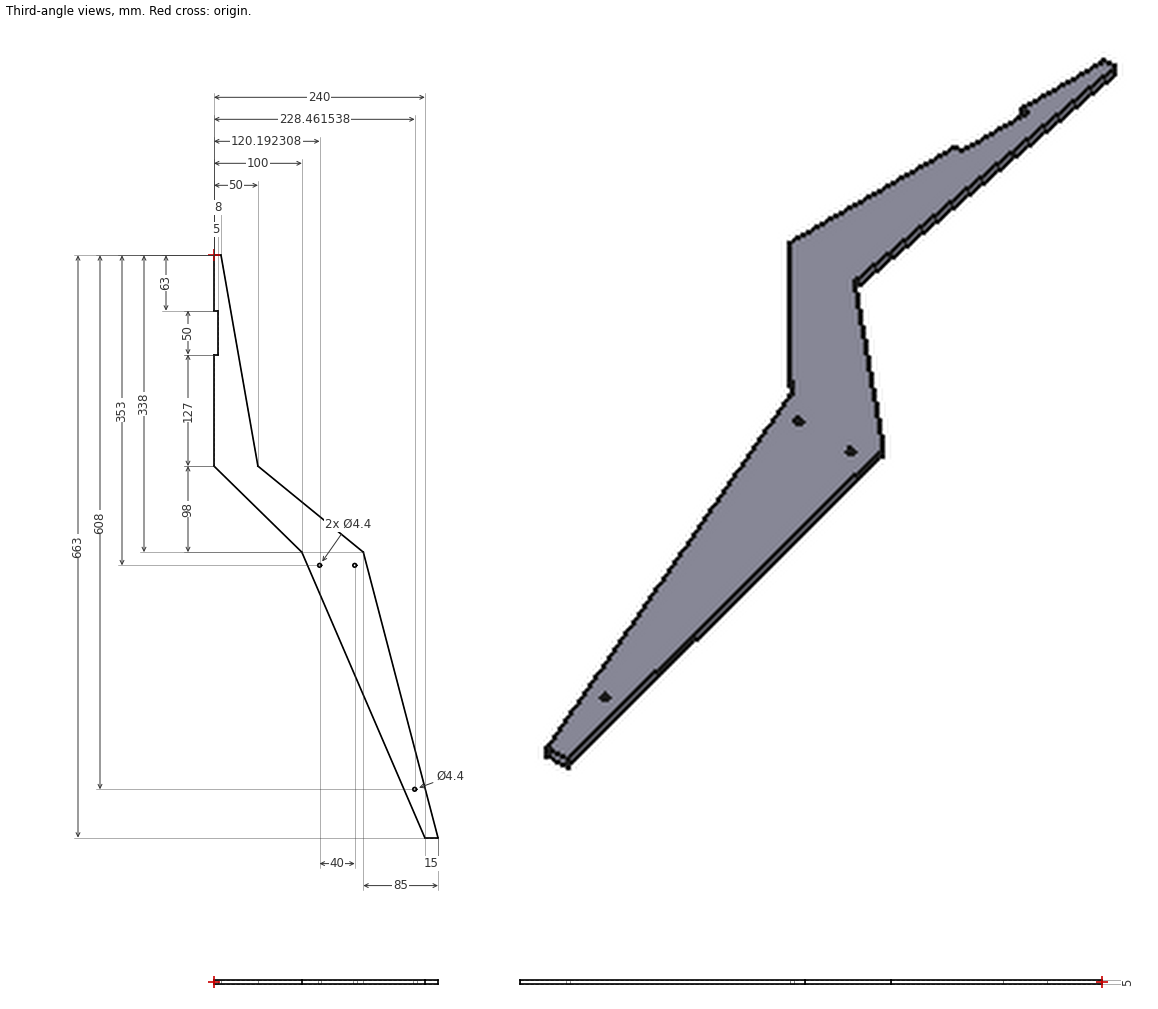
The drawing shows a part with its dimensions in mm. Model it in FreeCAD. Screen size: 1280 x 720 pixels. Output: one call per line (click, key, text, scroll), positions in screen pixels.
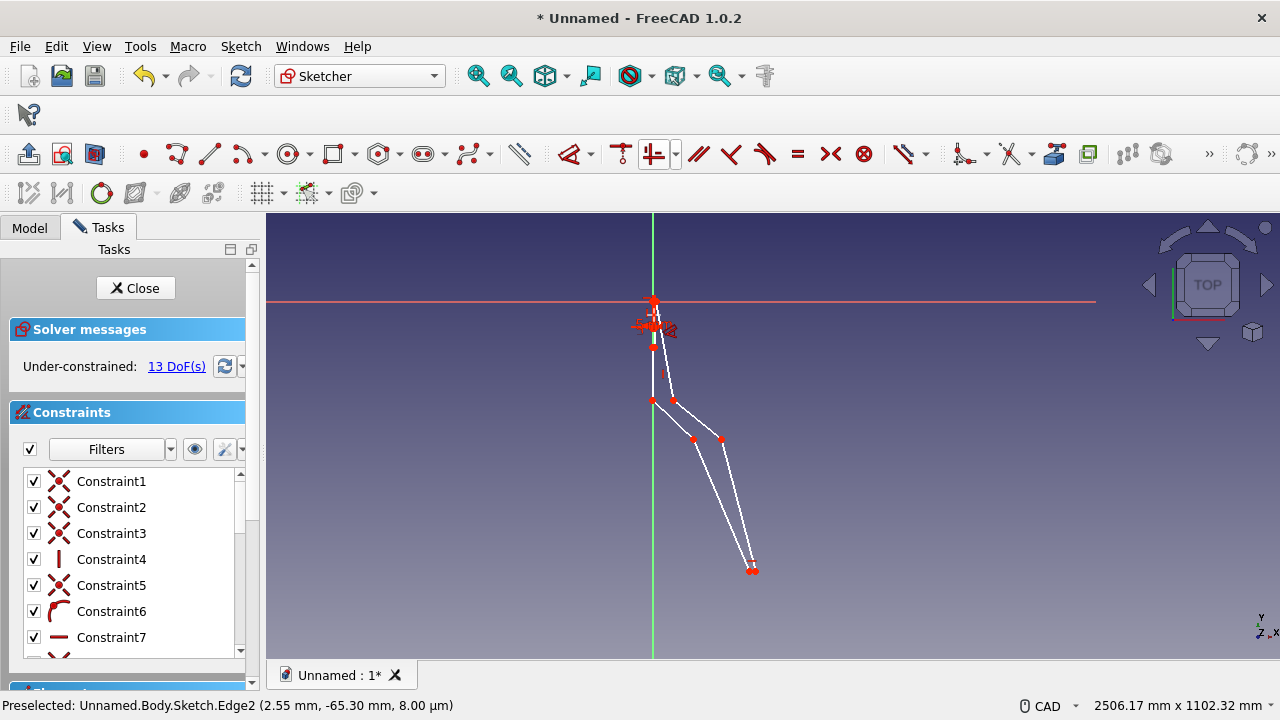
scroll(655, 302, up, 14)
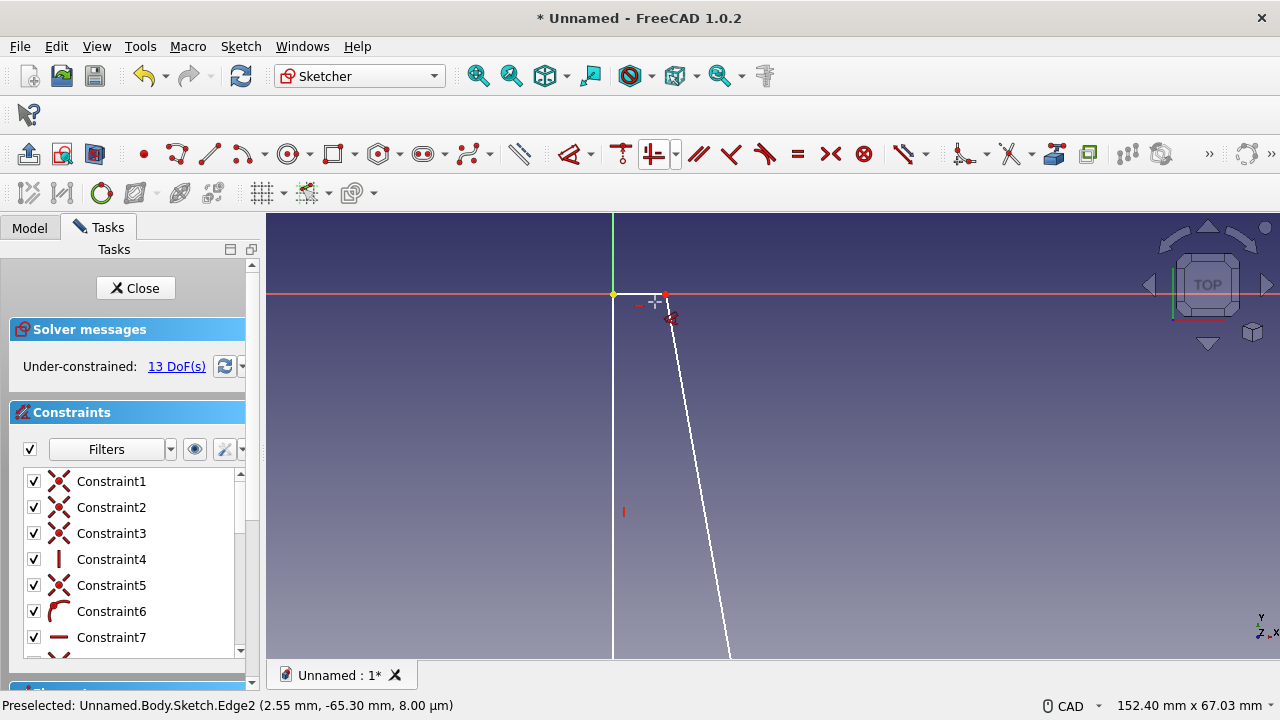
click(650, 294)
click(640, 260)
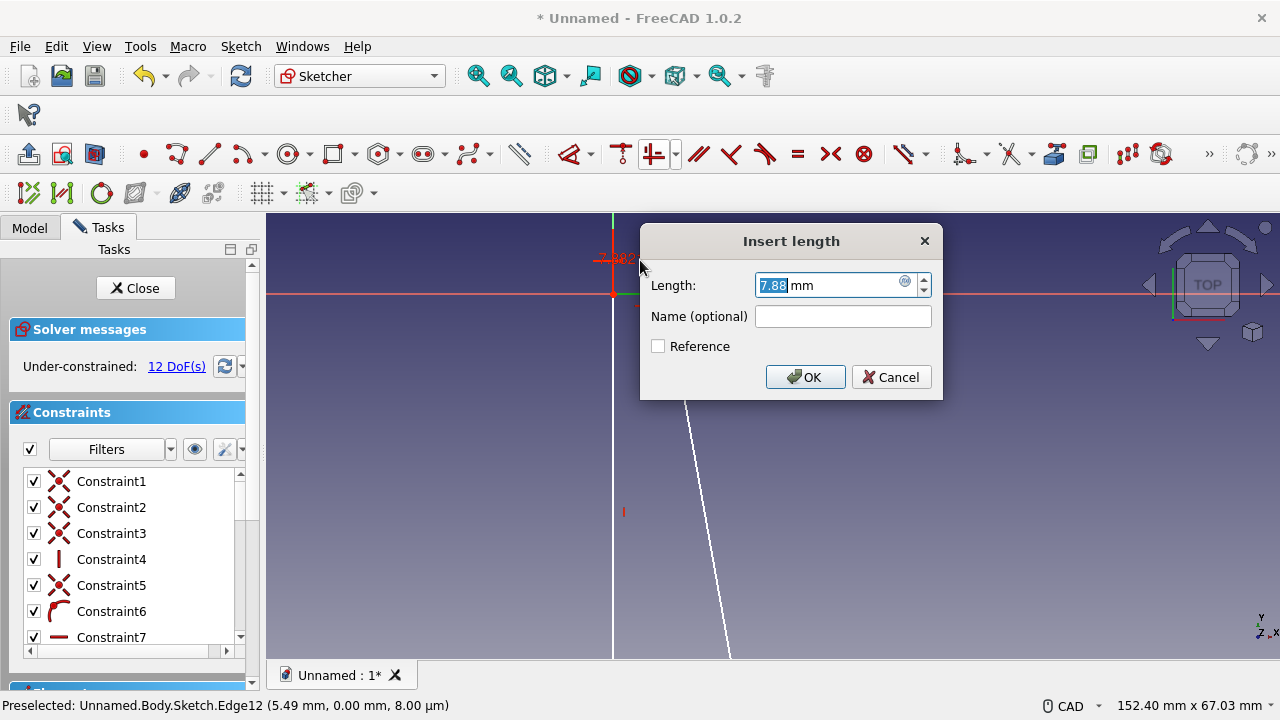
text(8)
key(Return)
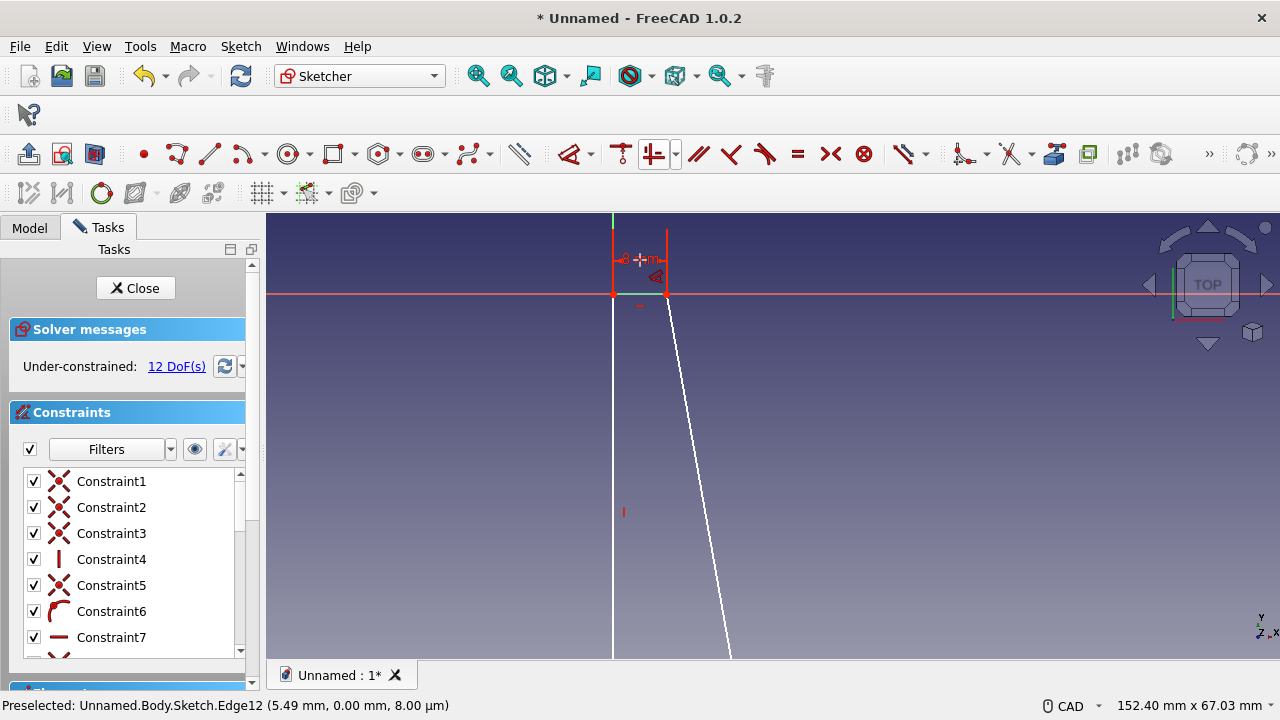
scroll(655, 302, down, 14)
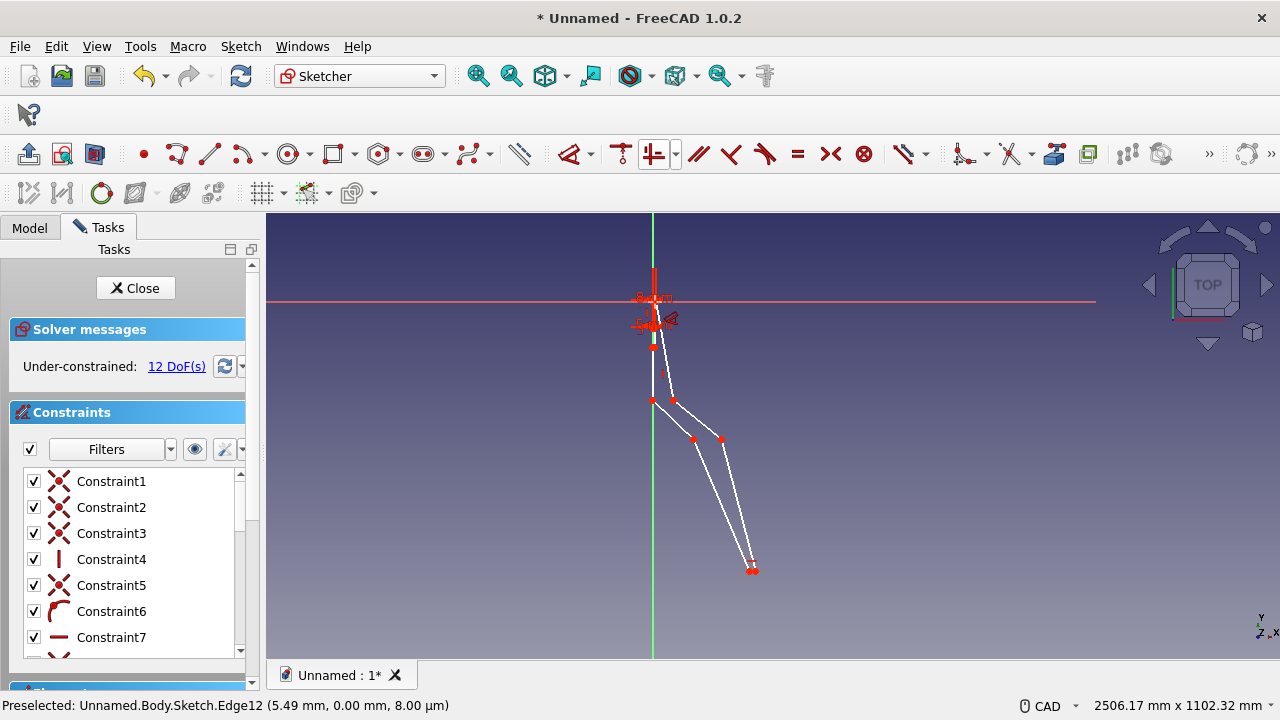
scroll(653, 310, up, 6)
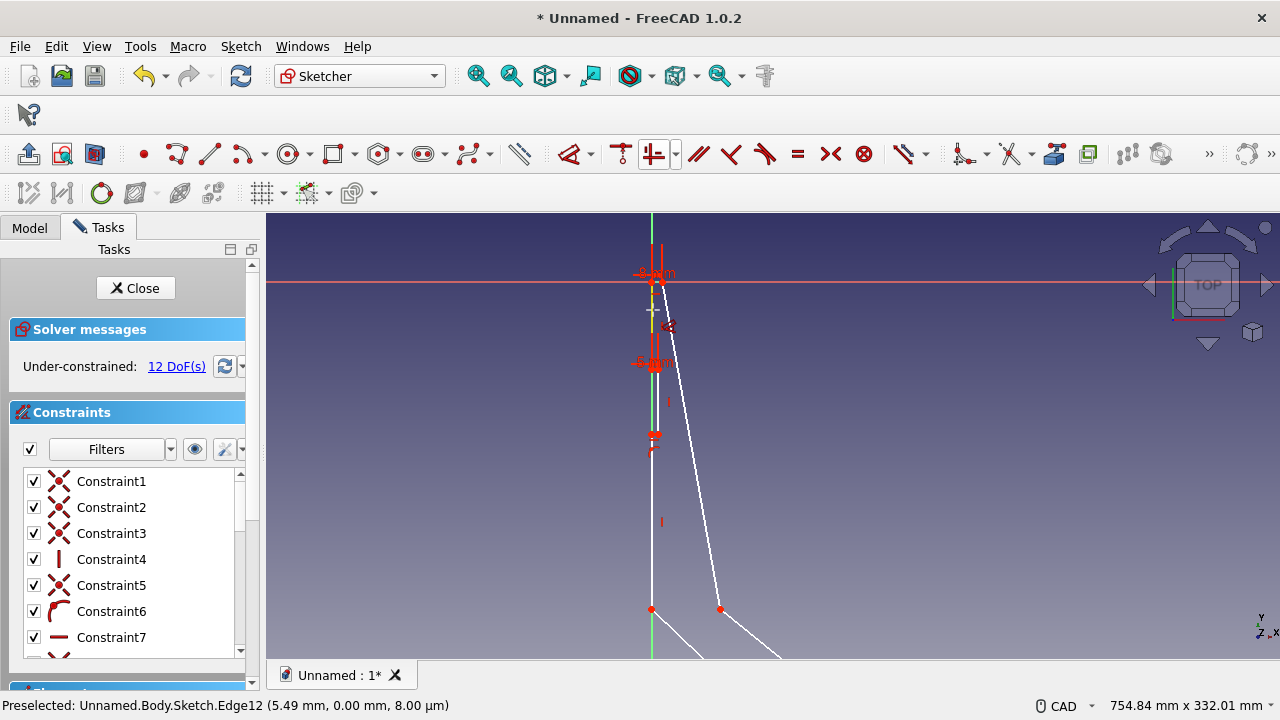
click(652, 308)
click(618, 326)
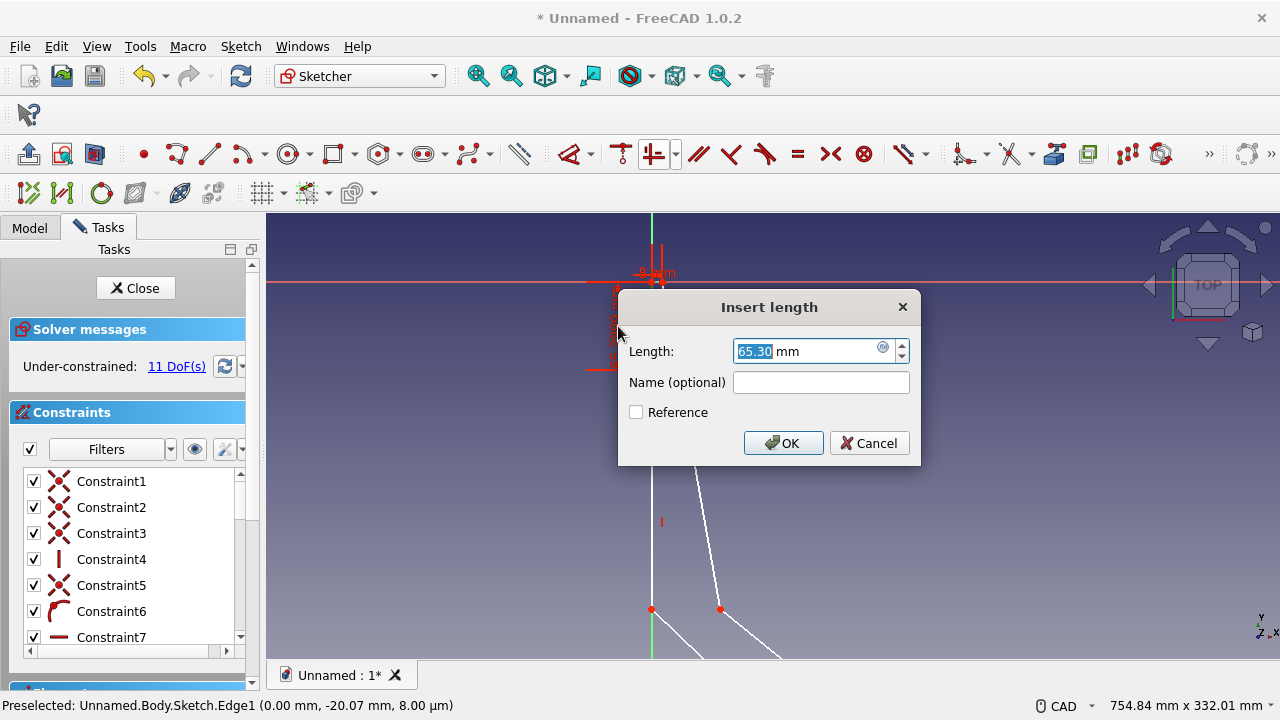
text(63)
key(Return)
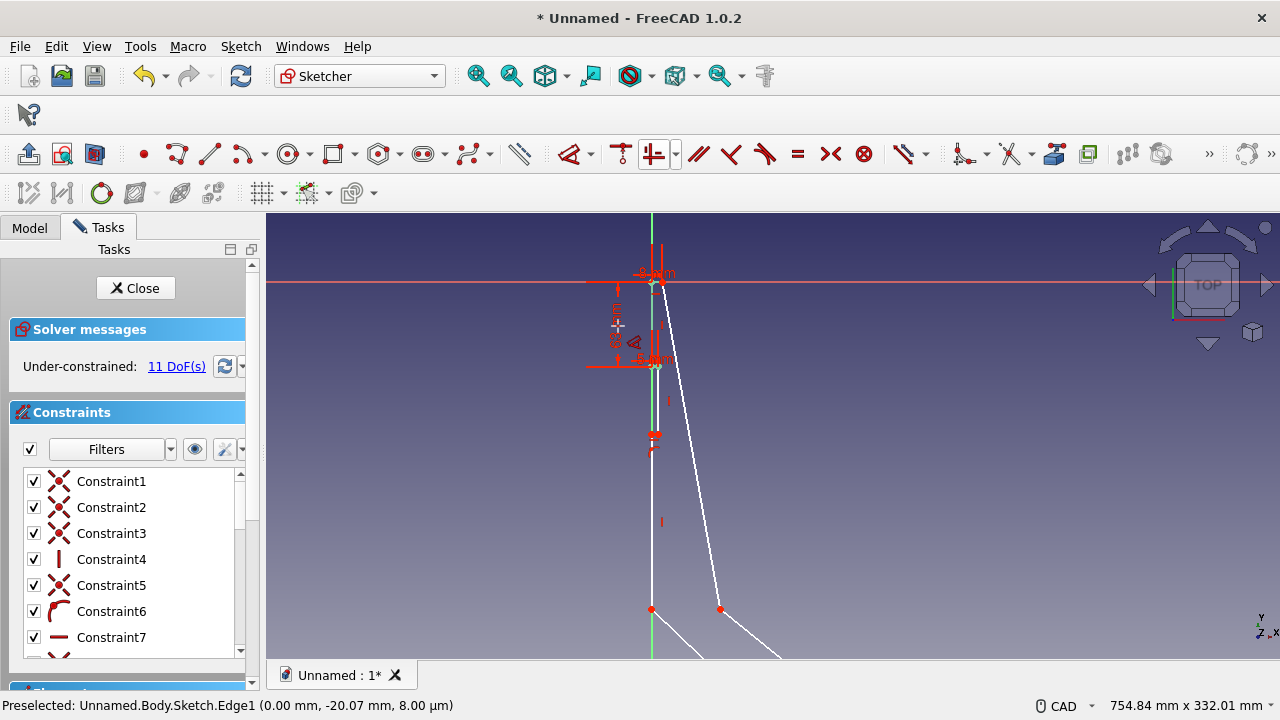
scroll(658, 387, up, 4)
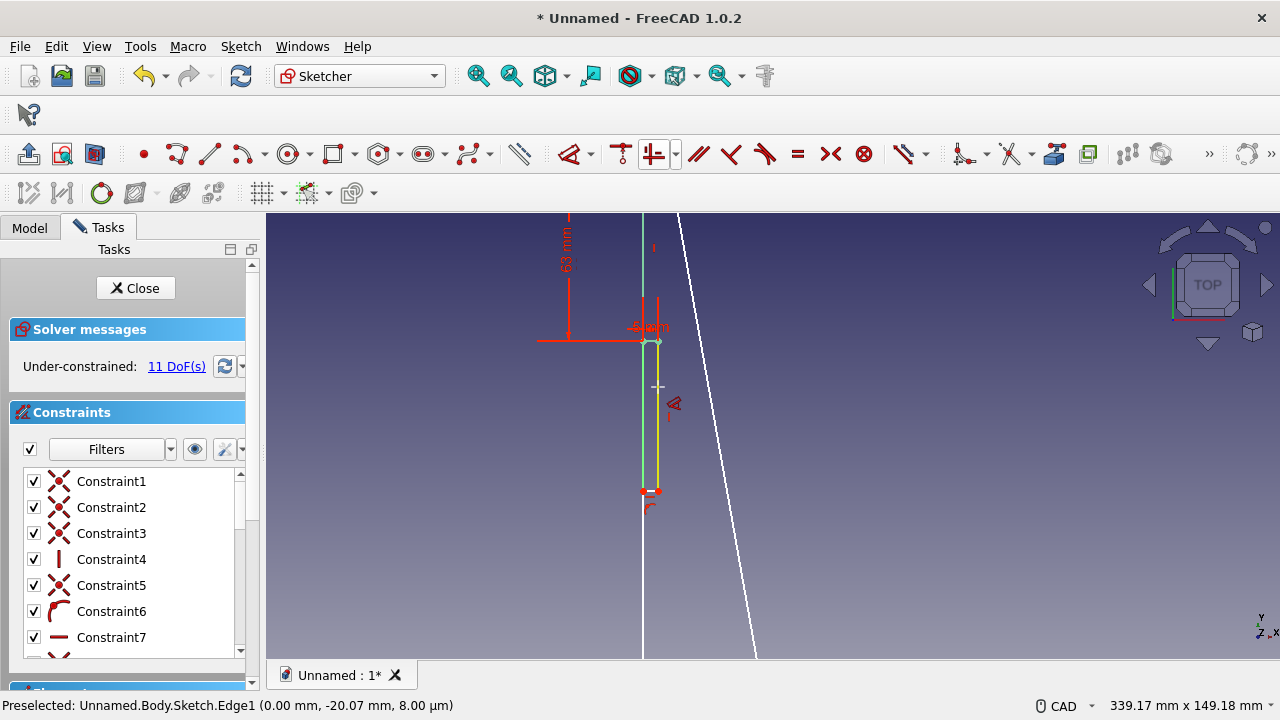
click(658, 386)
click(624, 416)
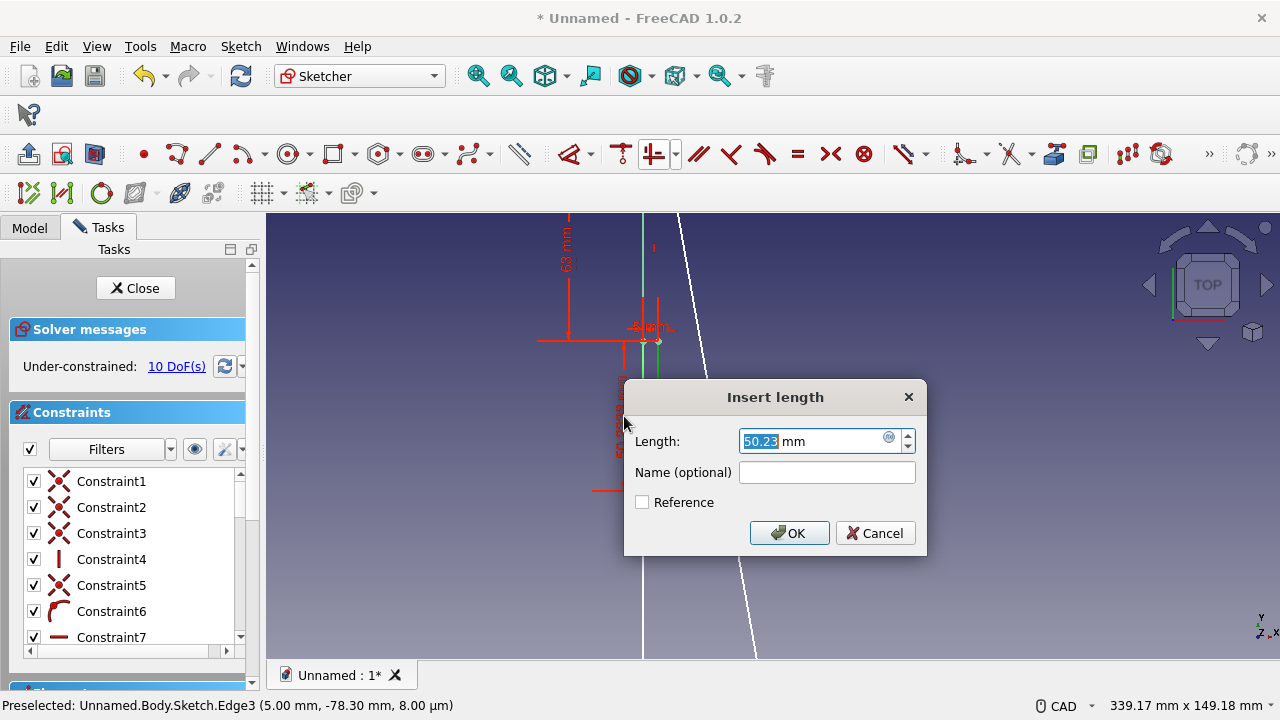
text(50)
key(Return)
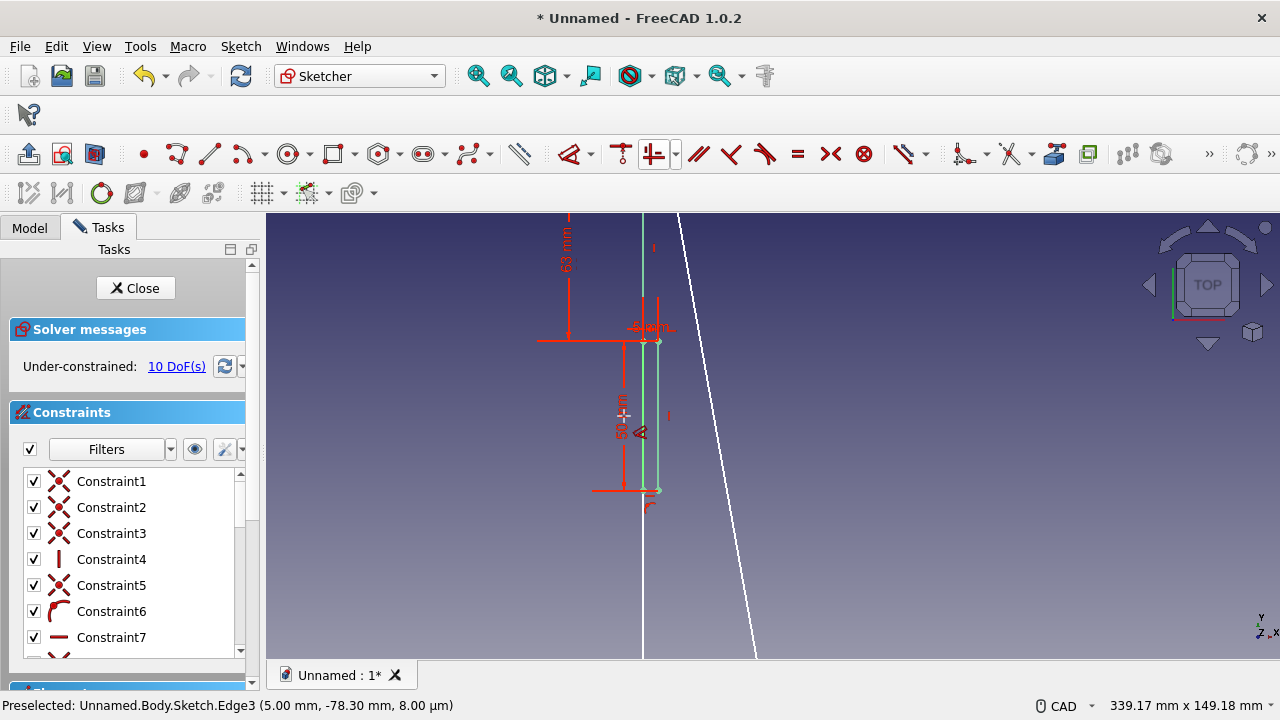
scroll(654, 325, down, 10)